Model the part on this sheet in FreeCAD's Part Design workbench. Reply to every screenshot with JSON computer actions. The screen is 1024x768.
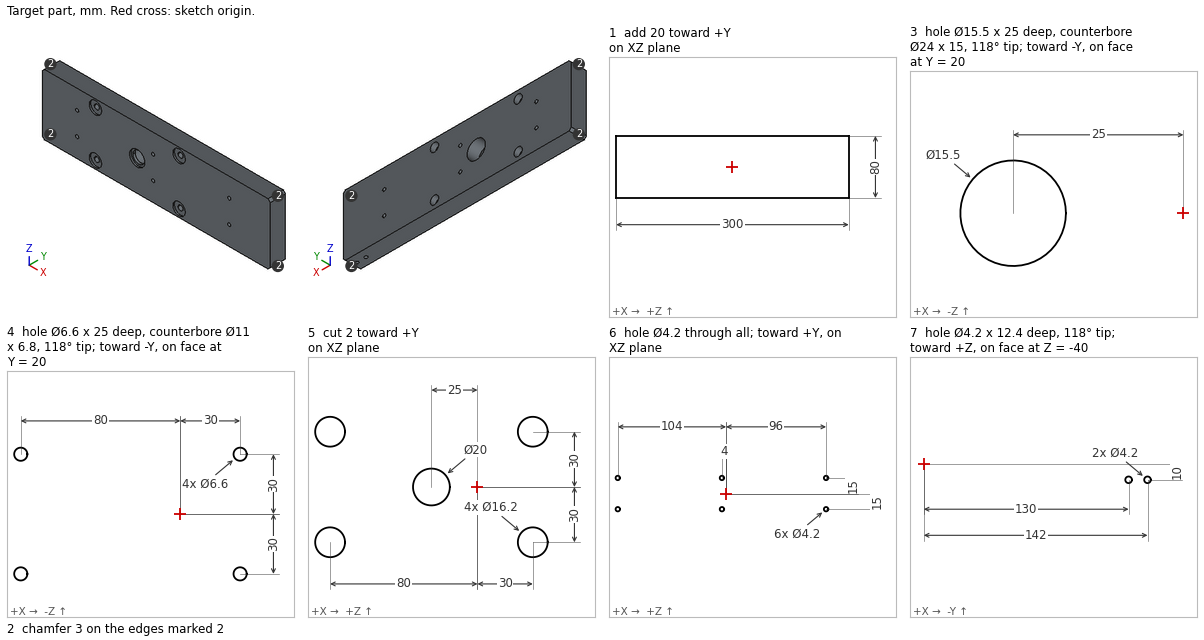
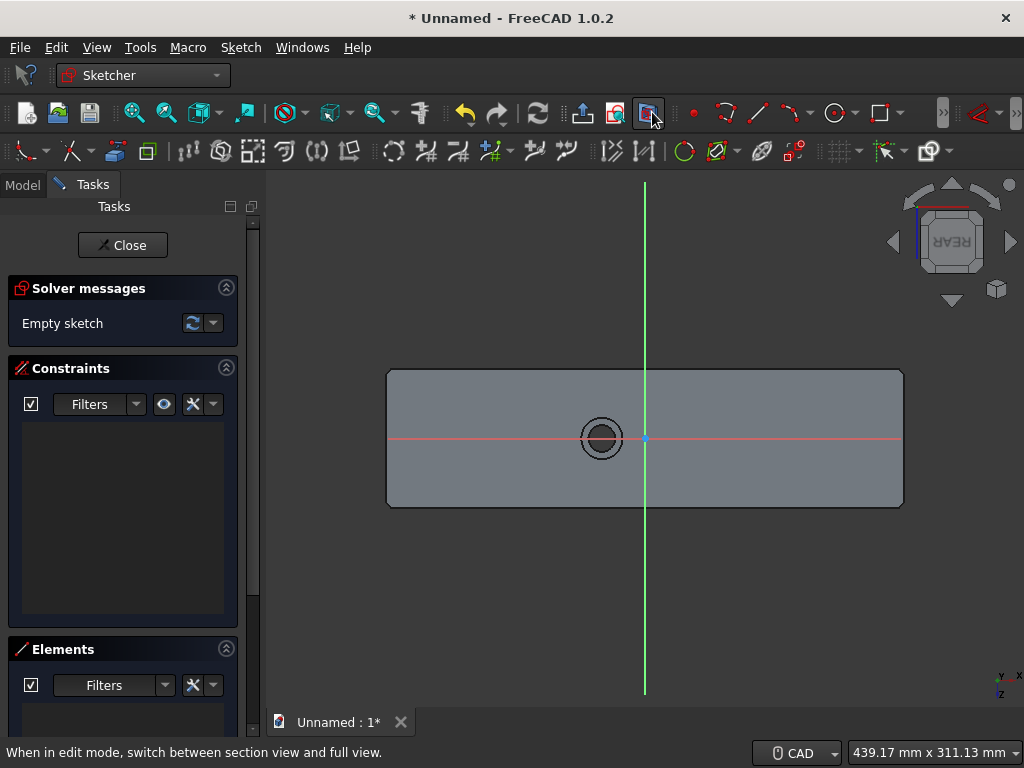
{"action": "scroll", "coordinate": [633, 438], "scroll_direction": "up", "scroll_amount": 3}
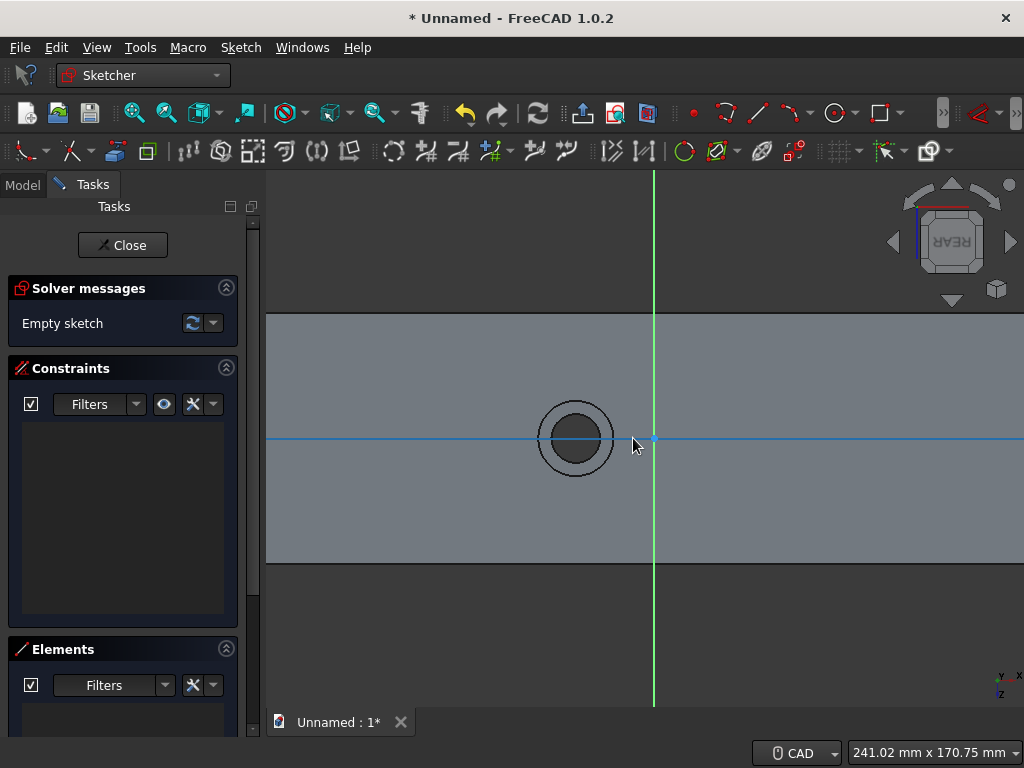
{"action": "left_click", "coordinate": [836, 114]}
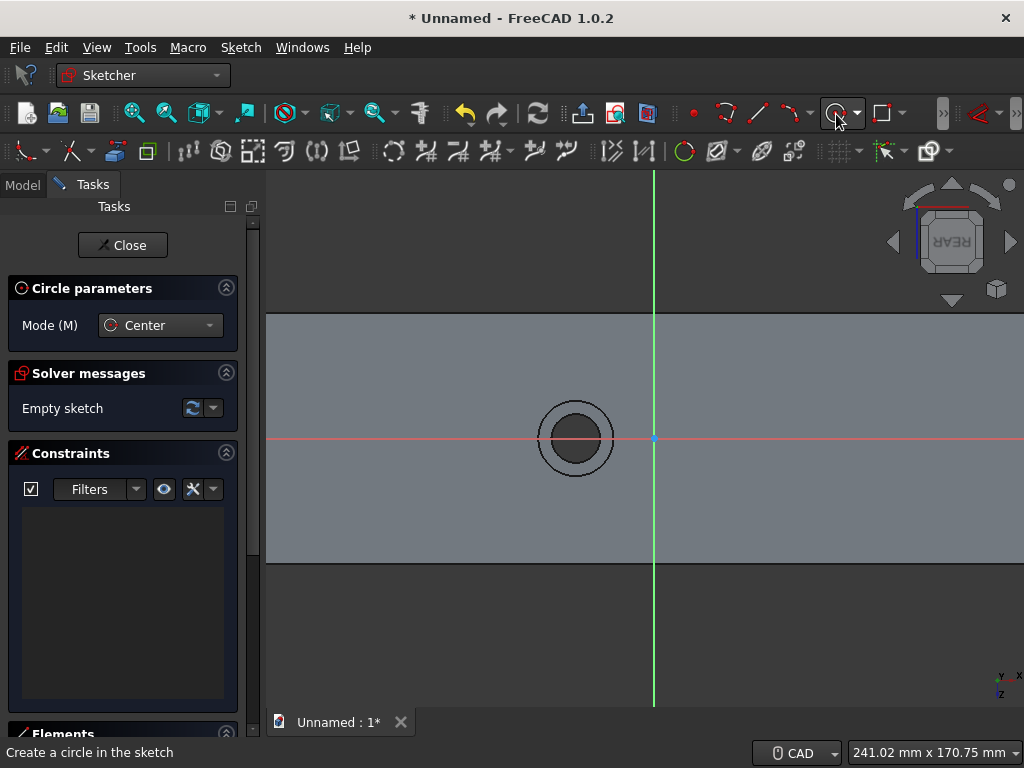
{"action": "scroll", "coordinate": [749, 344], "scroll_direction": "up", "scroll_amount": 4}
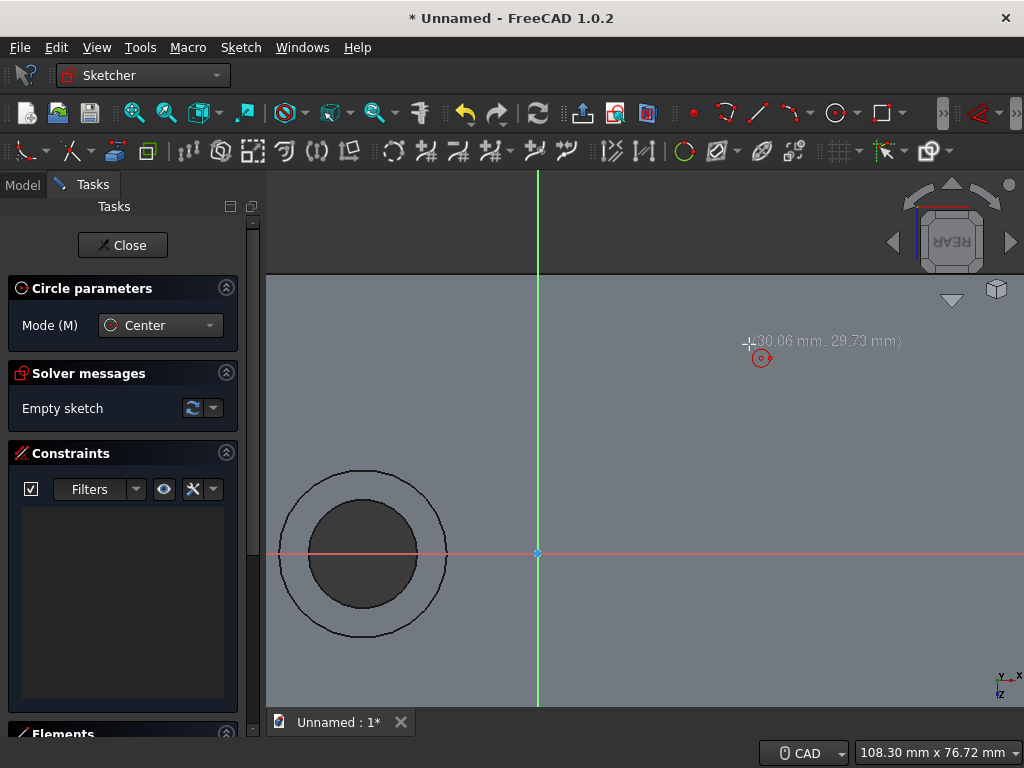
{"action": "left_click", "coordinate": [748, 344]}
{"action": "mouse_move", "coordinate": [764, 328]}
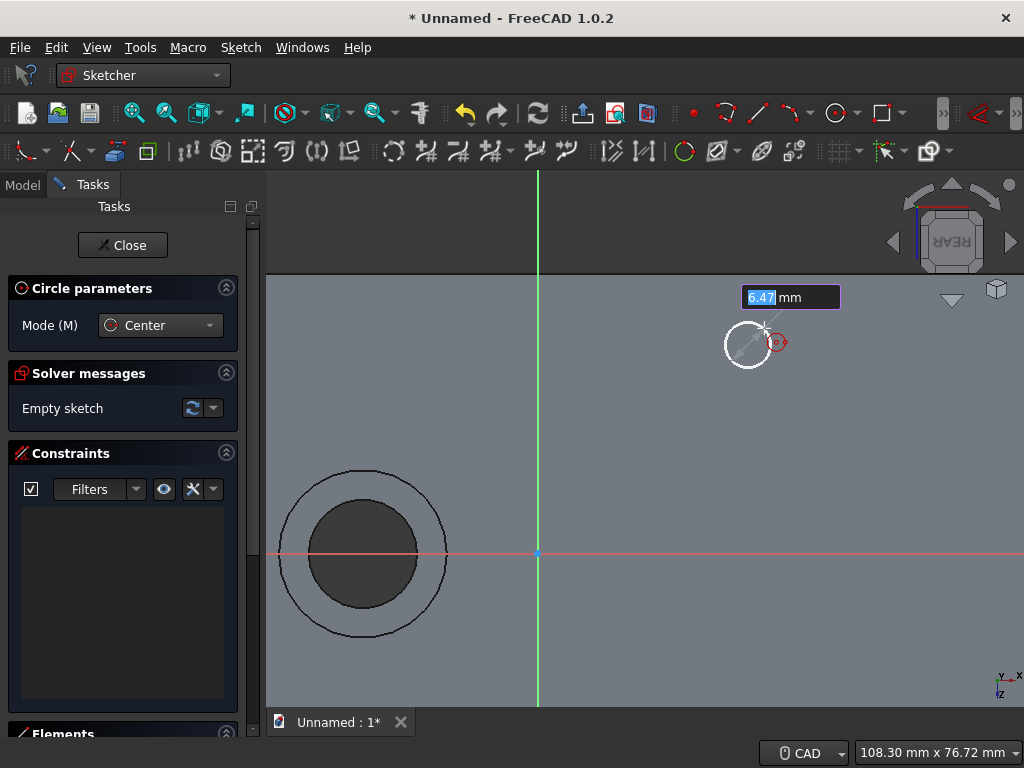
{"action": "type", "text": "6.6"}
{"action": "key", "text": "Return"}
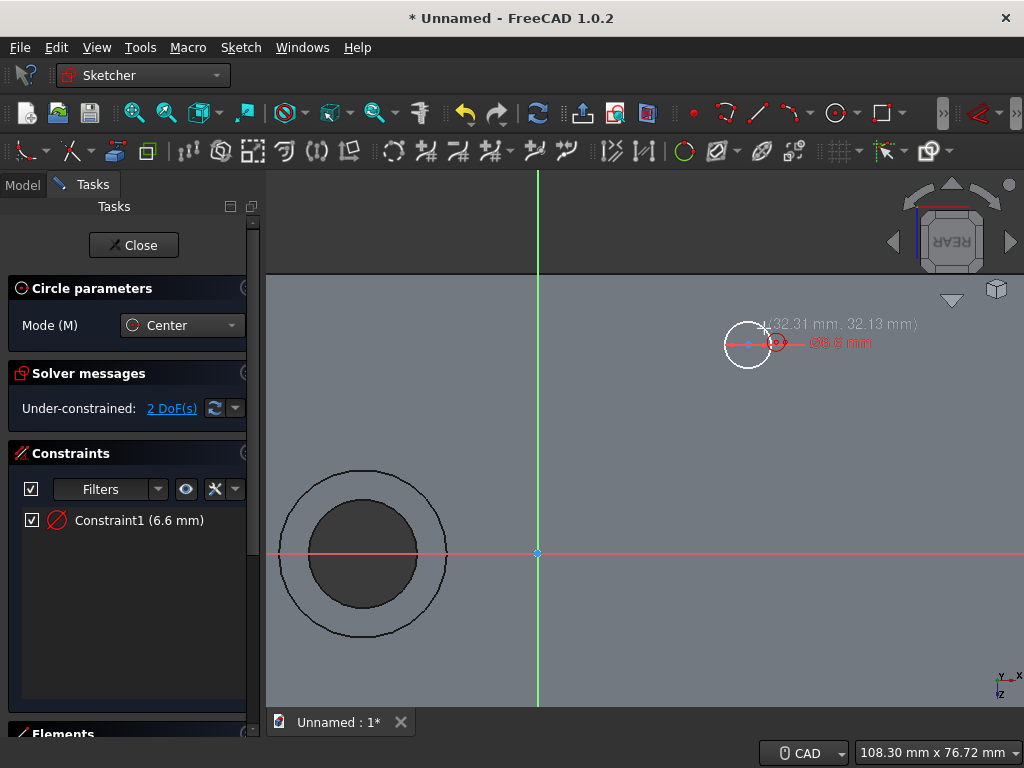
{"action": "scroll", "coordinate": [751, 344], "scroll_direction": "down", "scroll_amount": 4}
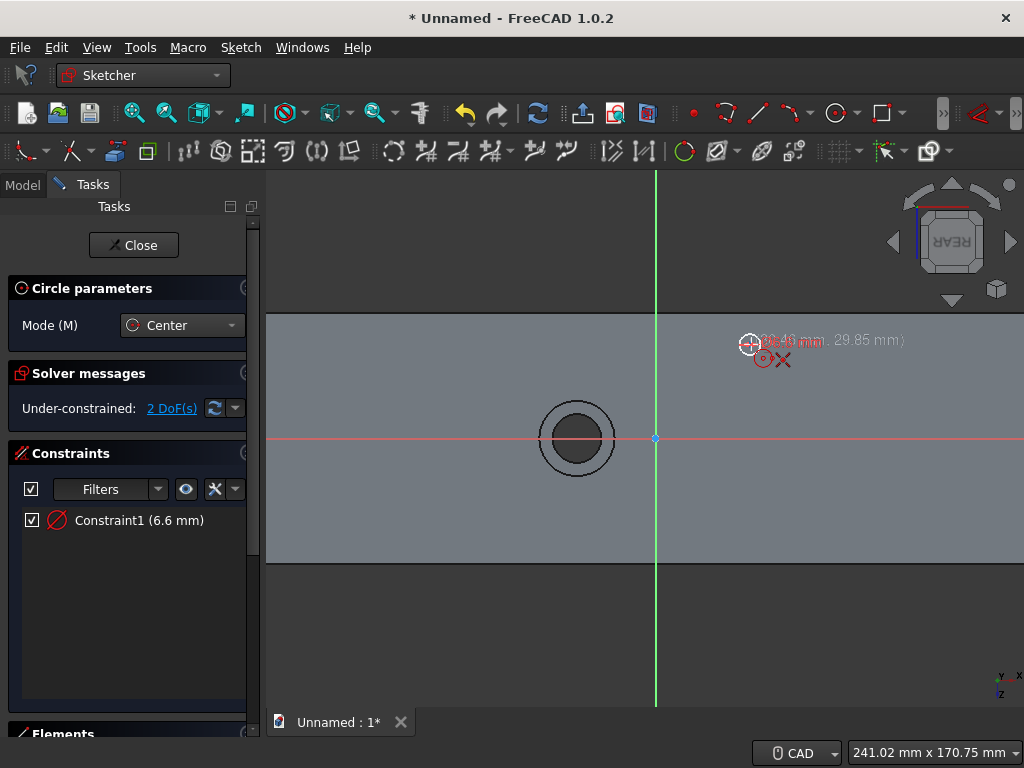
{"action": "scroll", "coordinate": [404, 344], "scroll_direction": "up", "scroll_amount": 4}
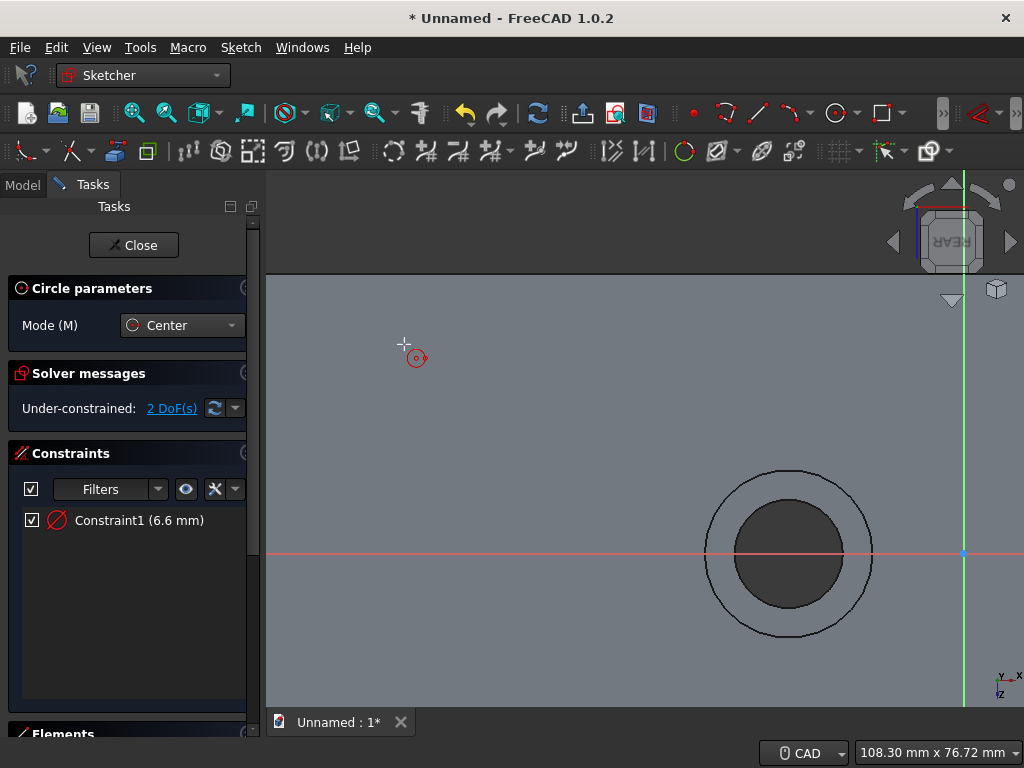
{"action": "left_click", "coordinate": [404, 344]}
{"action": "mouse_move", "coordinate": [420, 328]}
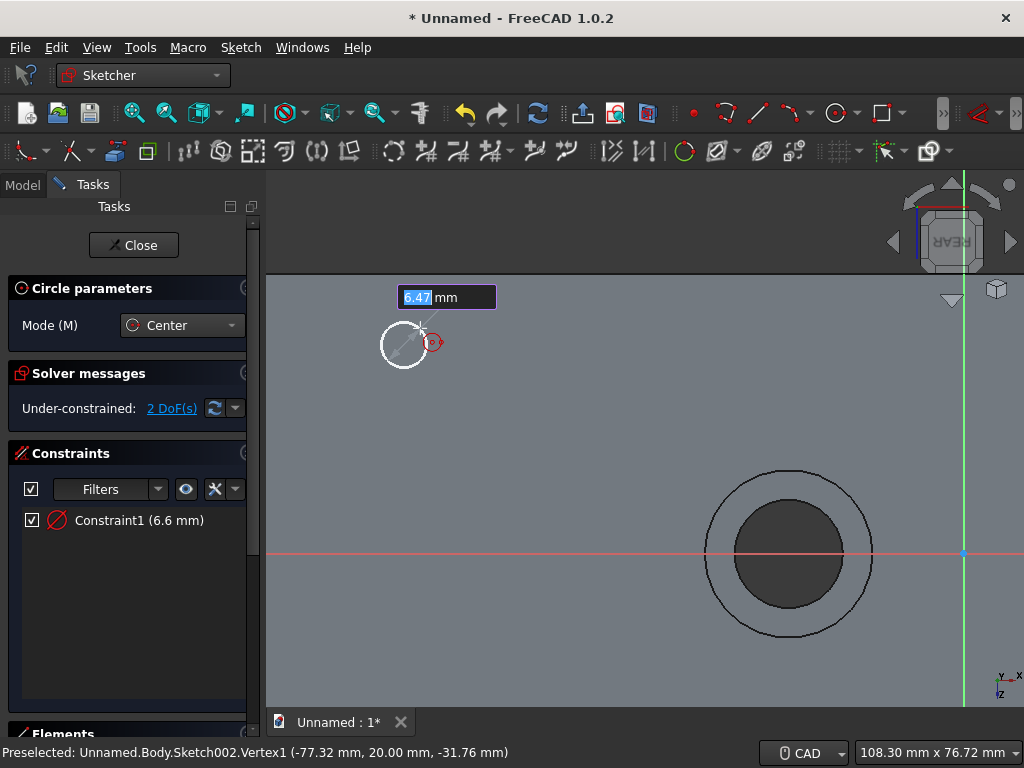
{"action": "type", "text": "6.6"}
{"action": "key", "text": "Return"}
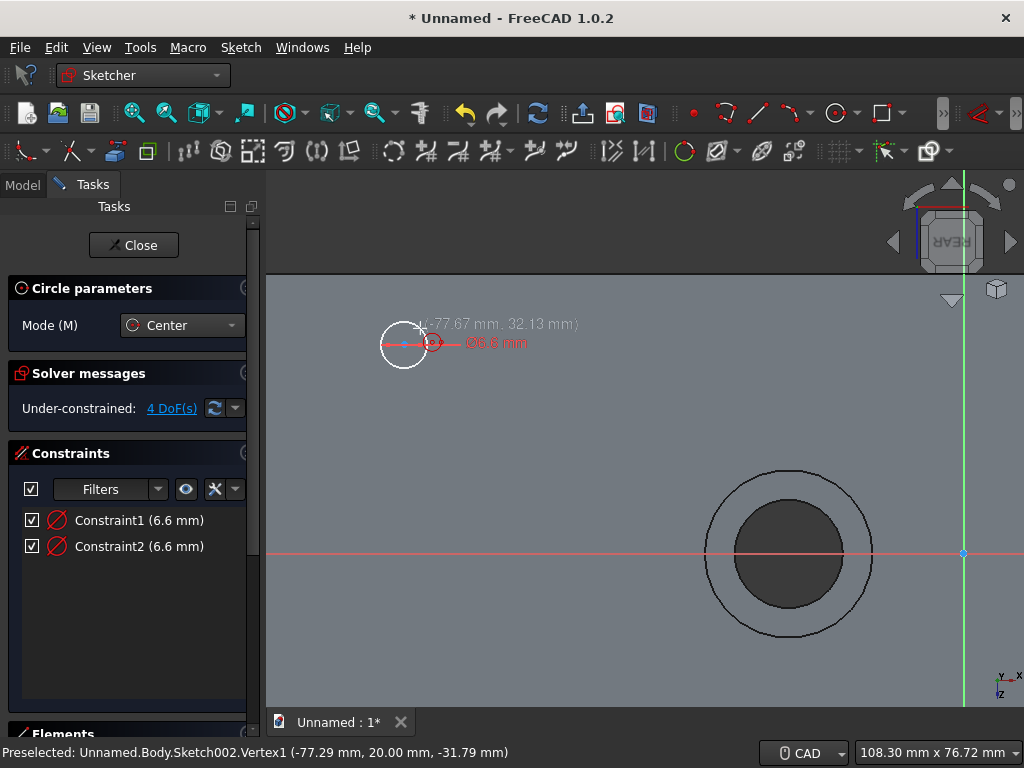
{"action": "scroll", "coordinate": [403, 344], "scroll_direction": "down", "scroll_amount": 4}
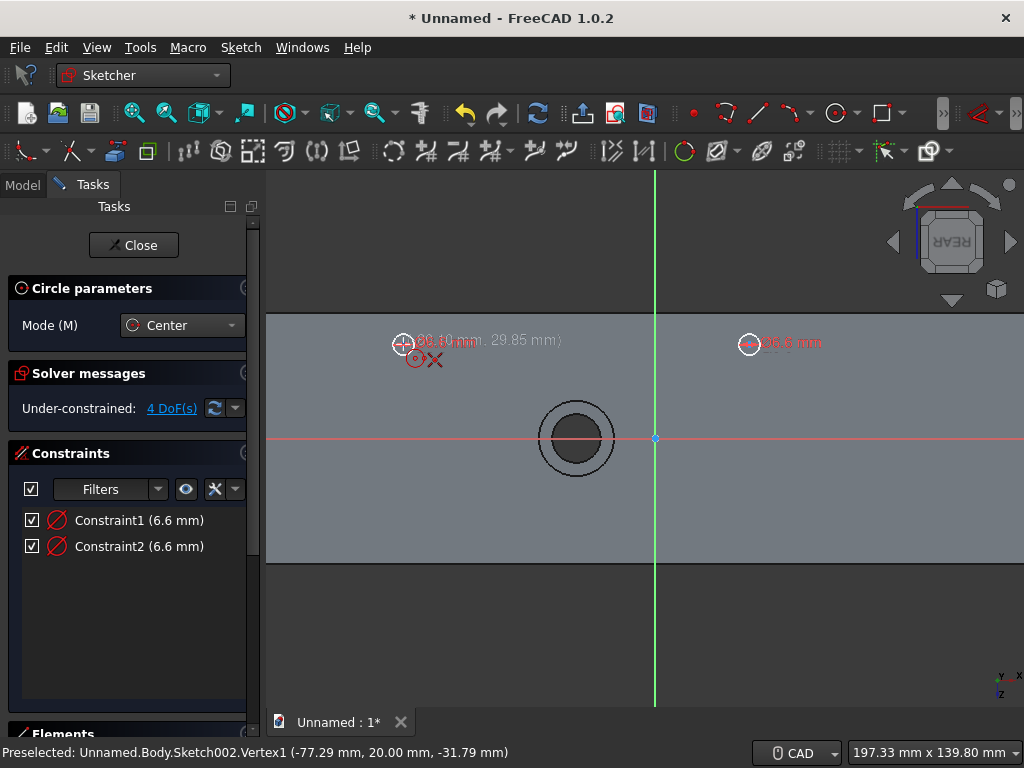
{"action": "scroll", "coordinate": [749, 533], "scroll_direction": "up", "scroll_amount": 4}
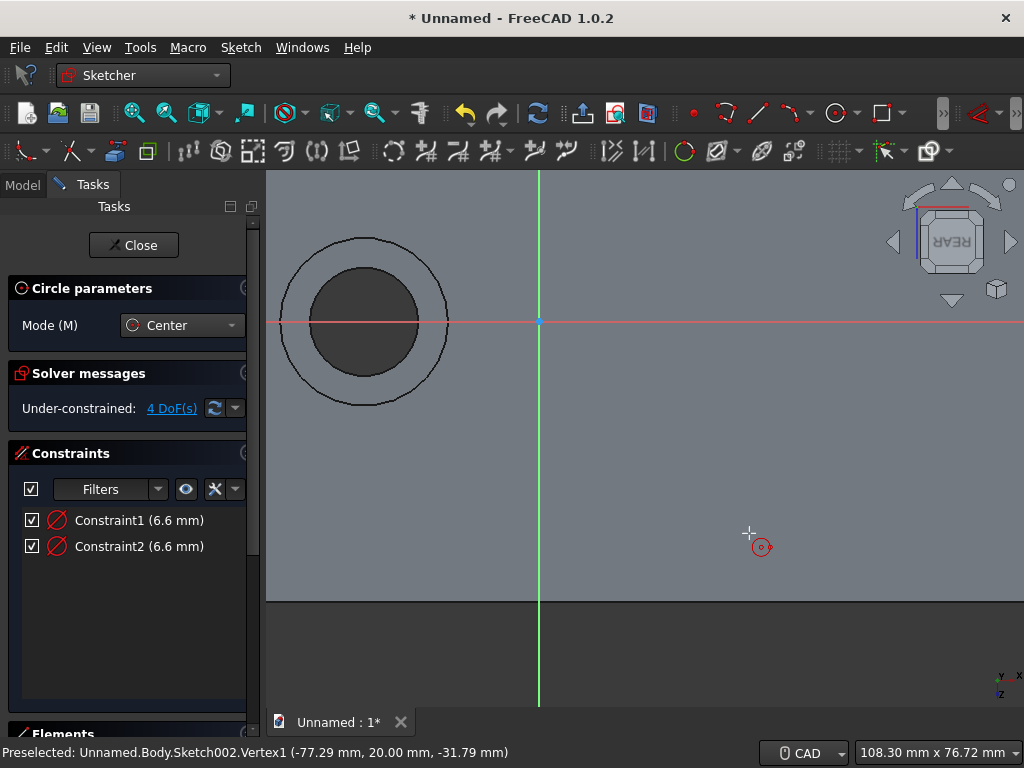
{"action": "left_click", "coordinate": [749, 532]}
{"action": "mouse_move", "coordinate": [765, 516]}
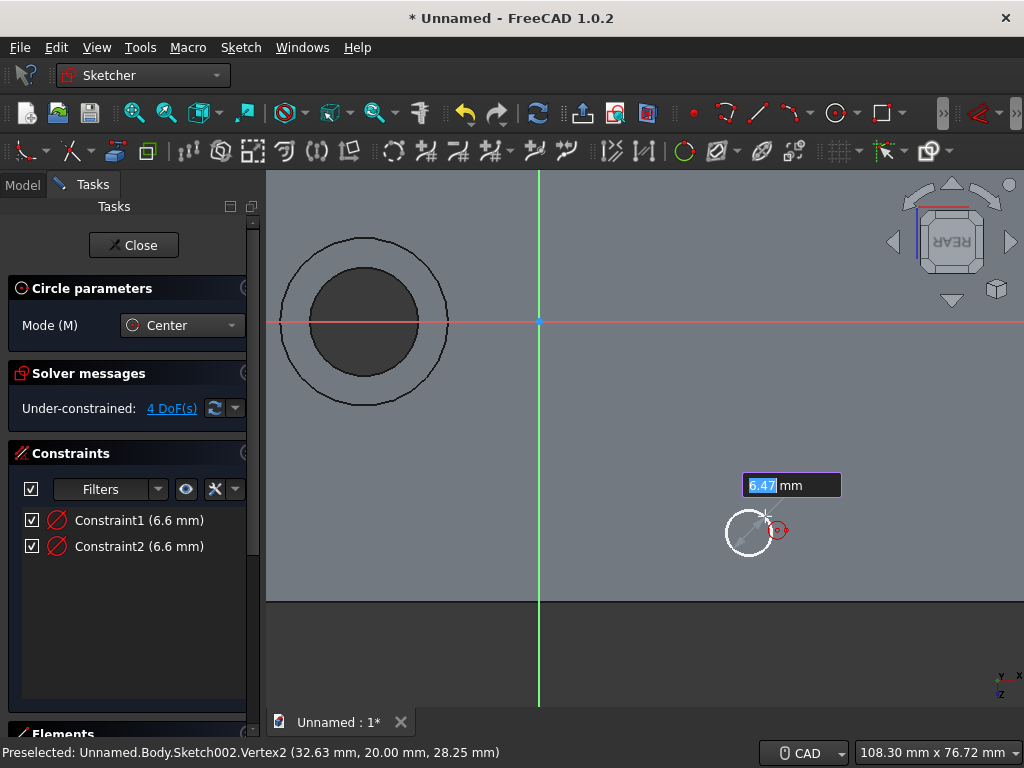
{"action": "type", "text": "6.6"}
{"action": "key", "text": "Return"}